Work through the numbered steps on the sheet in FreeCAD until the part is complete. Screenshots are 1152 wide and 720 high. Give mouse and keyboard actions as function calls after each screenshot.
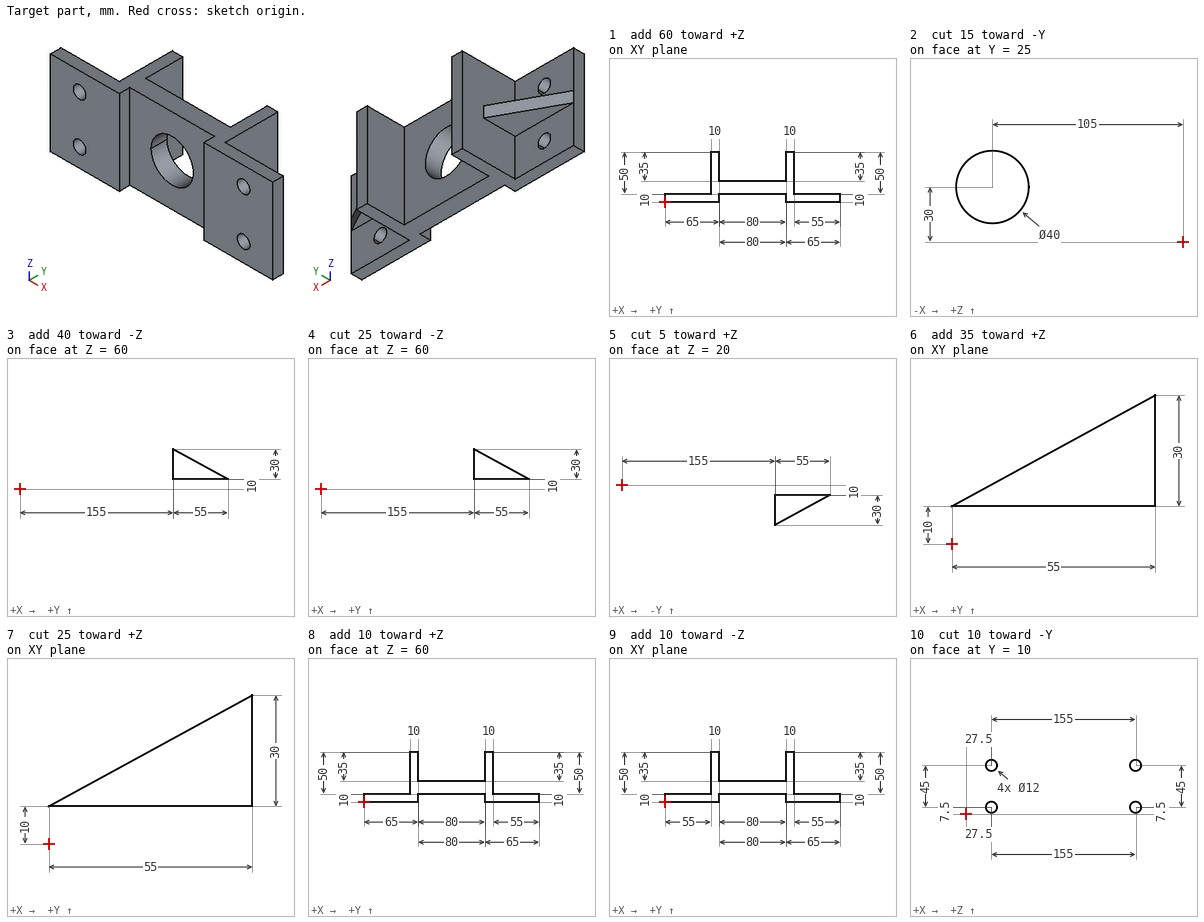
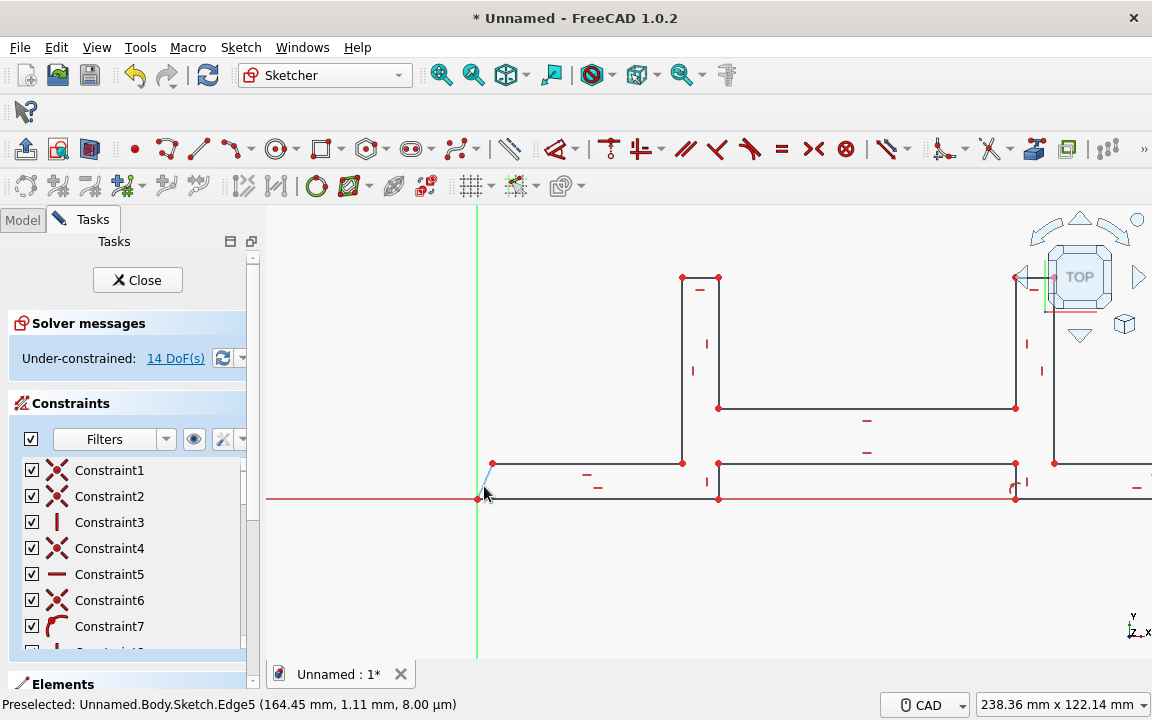
click(484, 485)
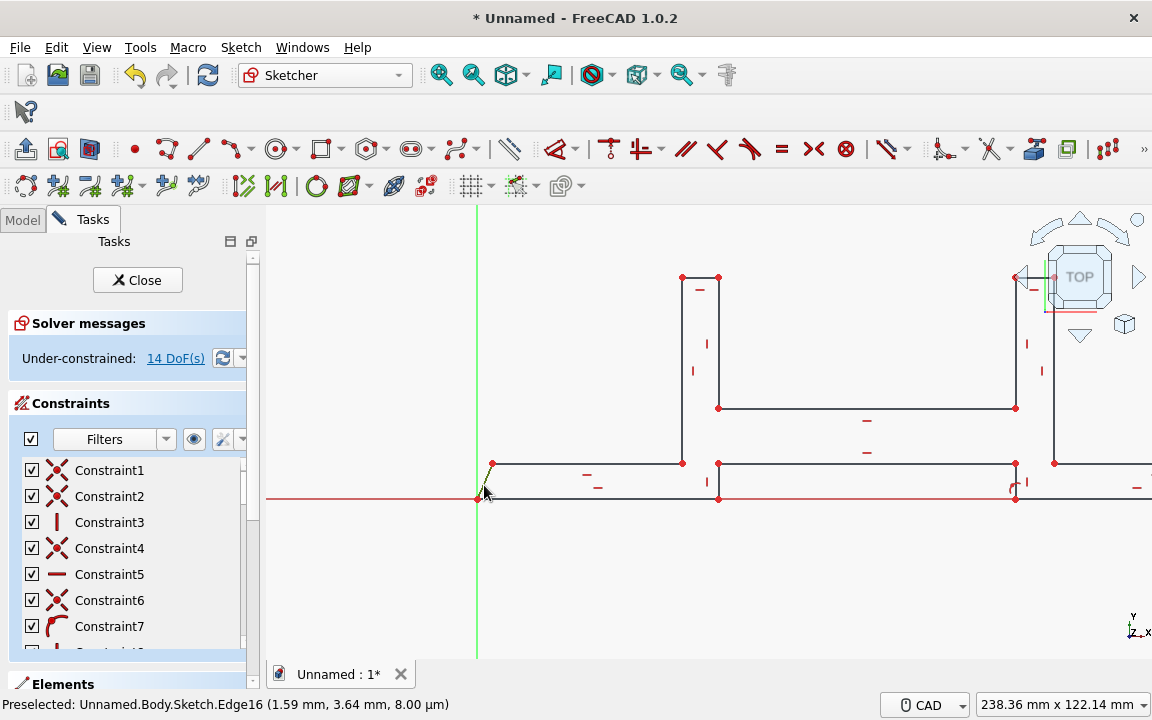
key(v)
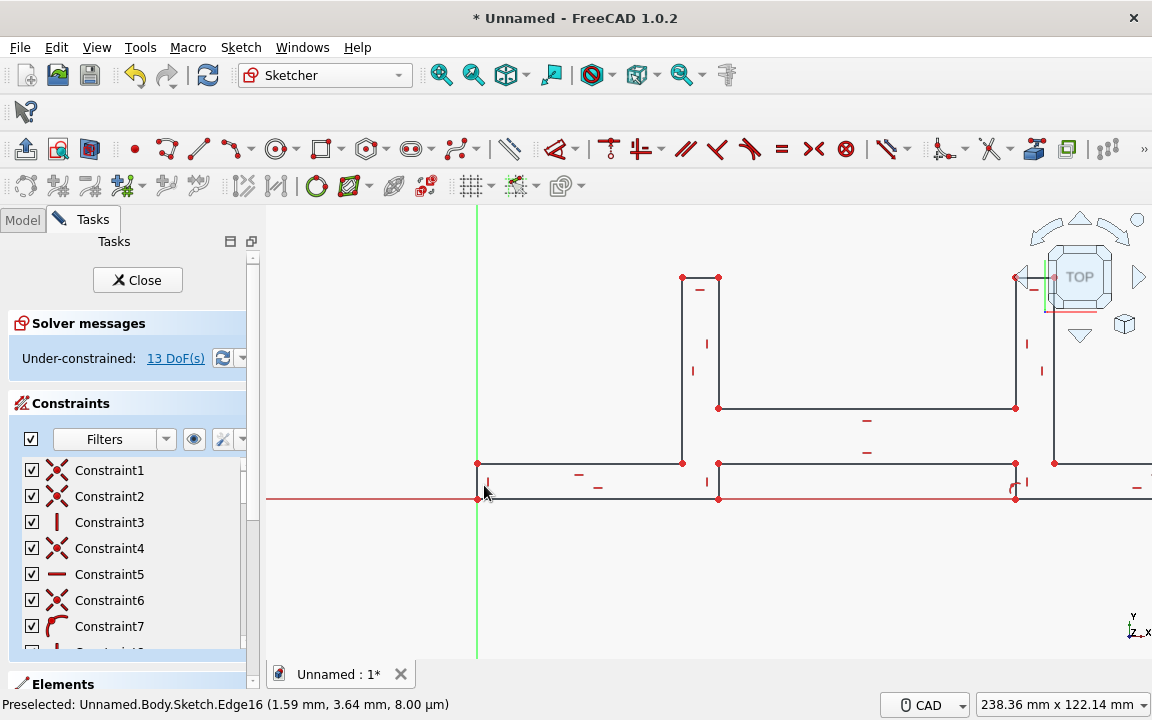
click(556, 150)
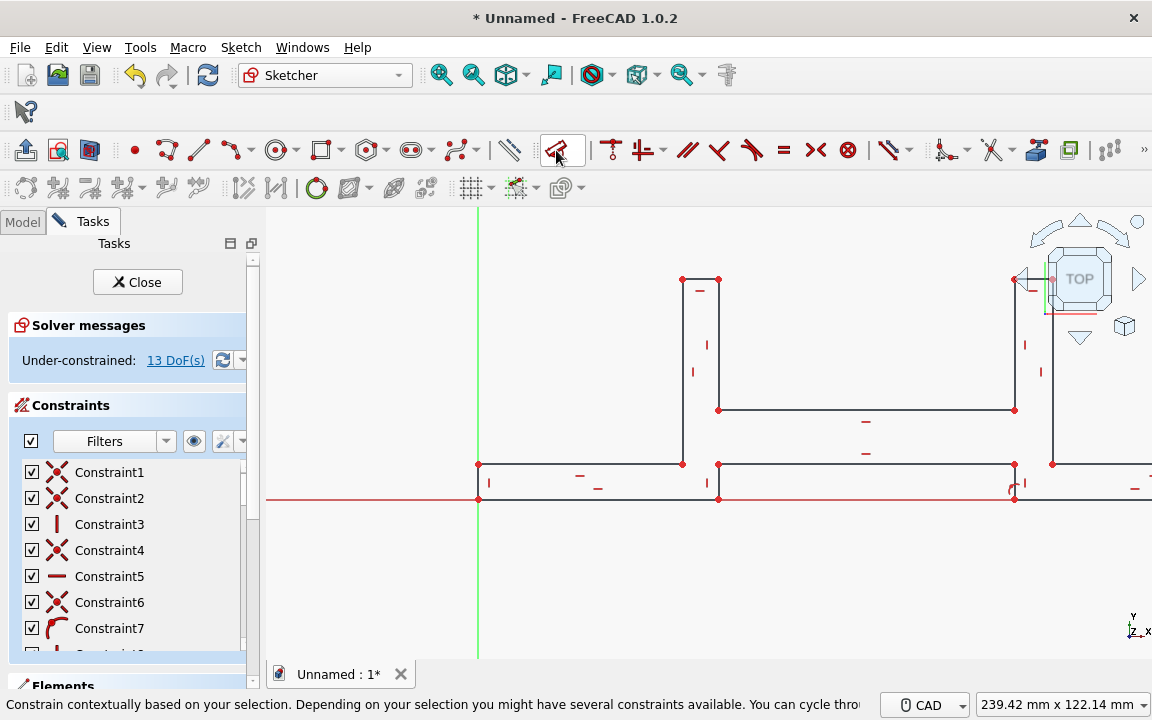
click(551, 500)
click(599, 534)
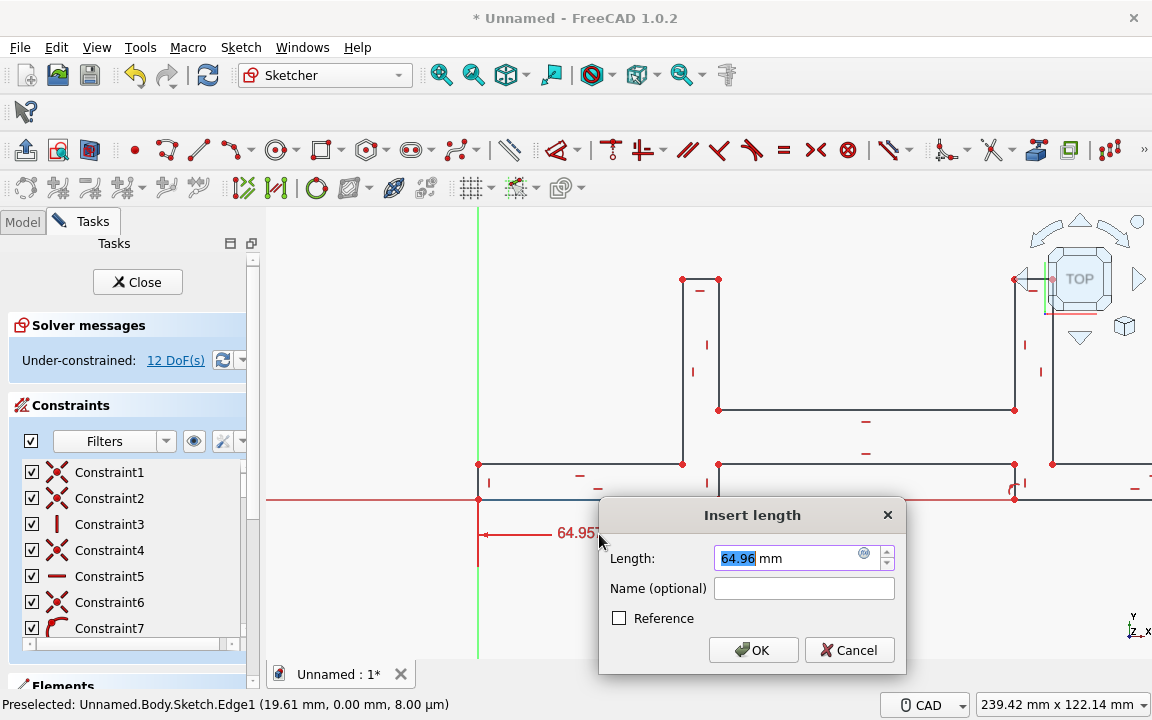
text(65)
key(Return)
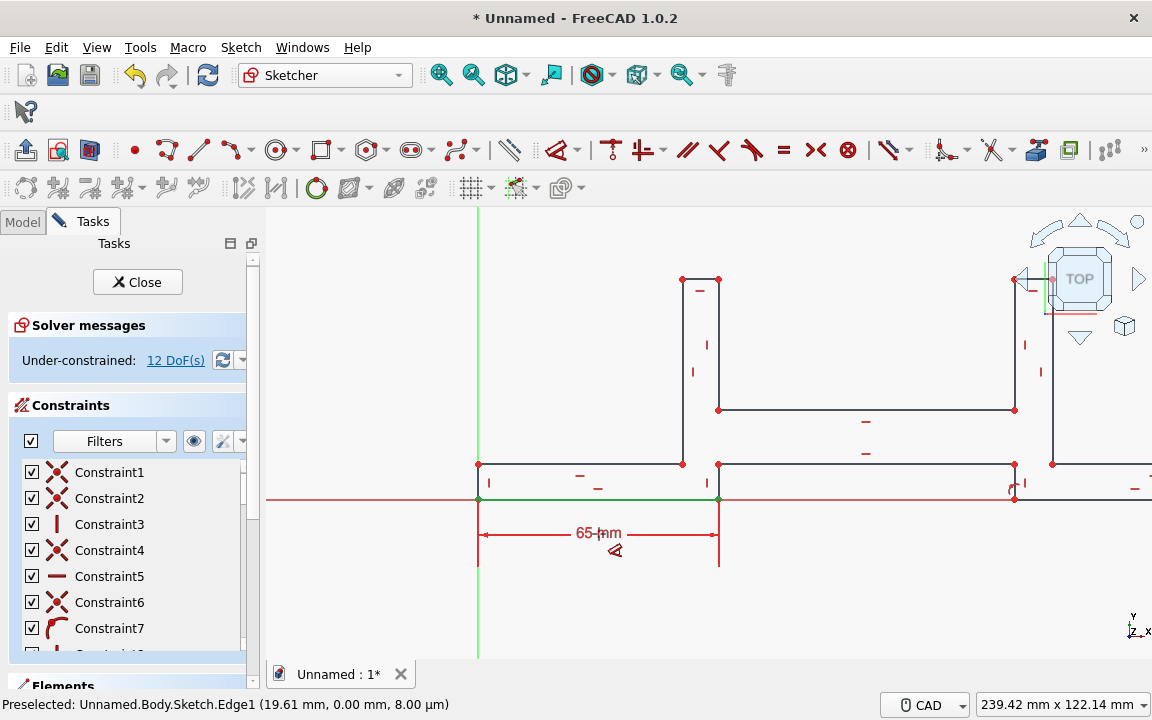
scroll(719, 489, up, 2)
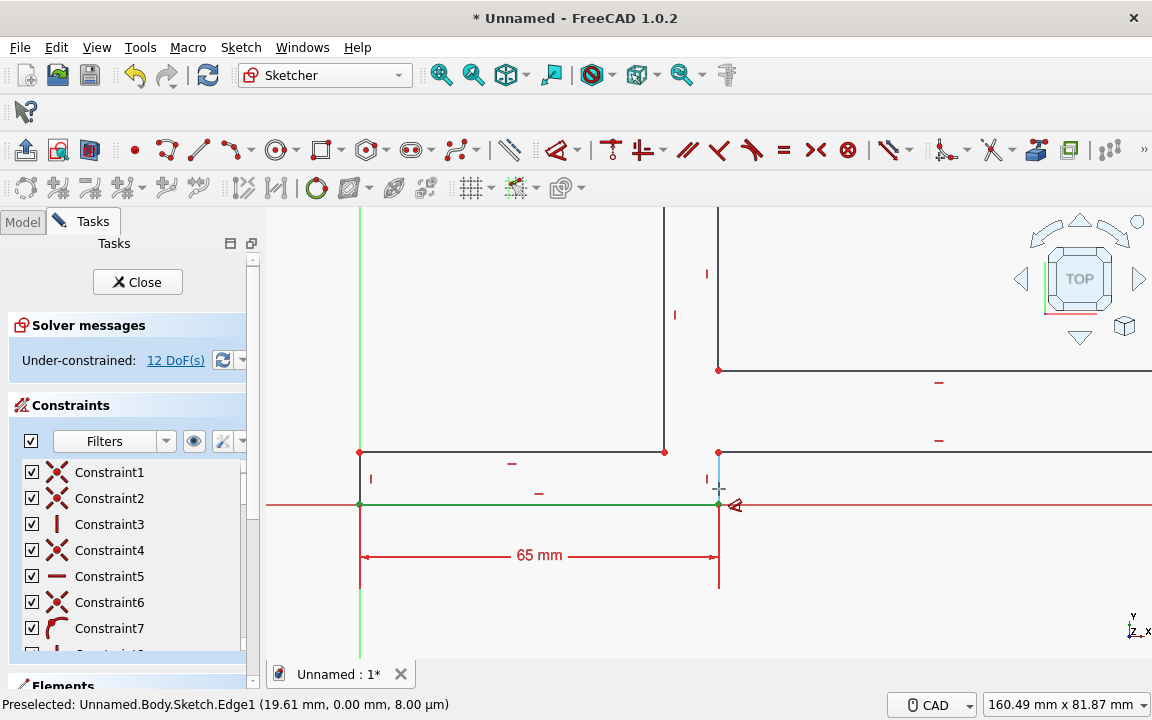
click(719, 489)
click(685, 479)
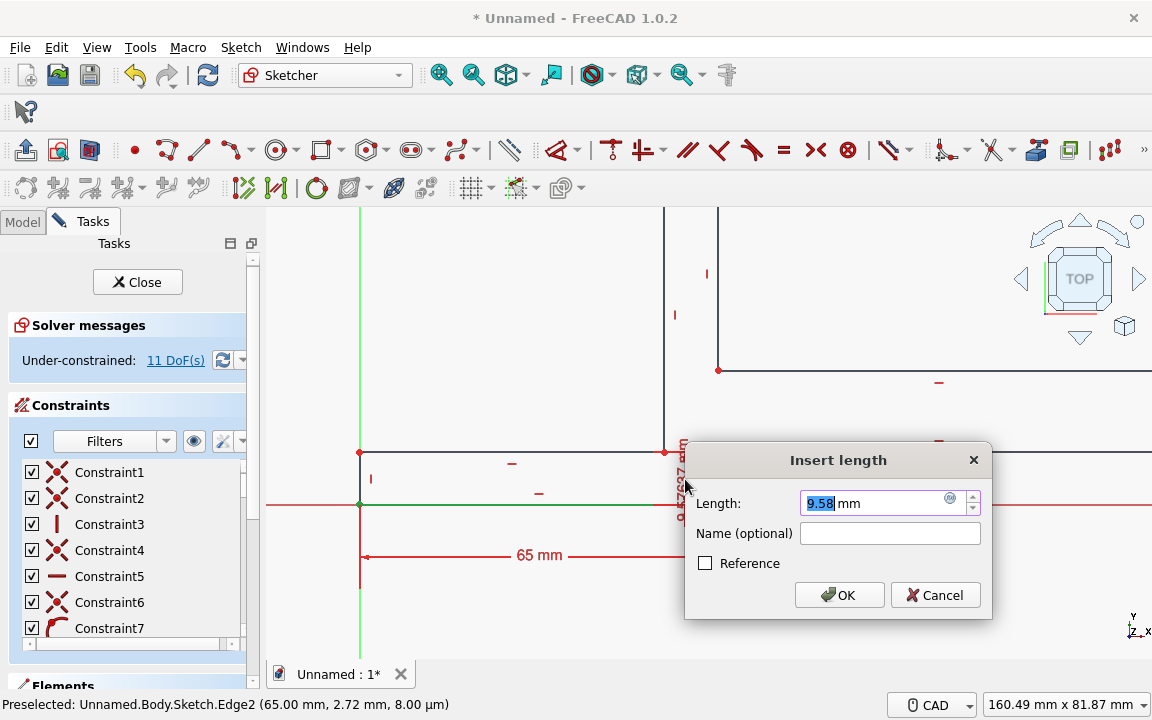
text(10)
key(Return)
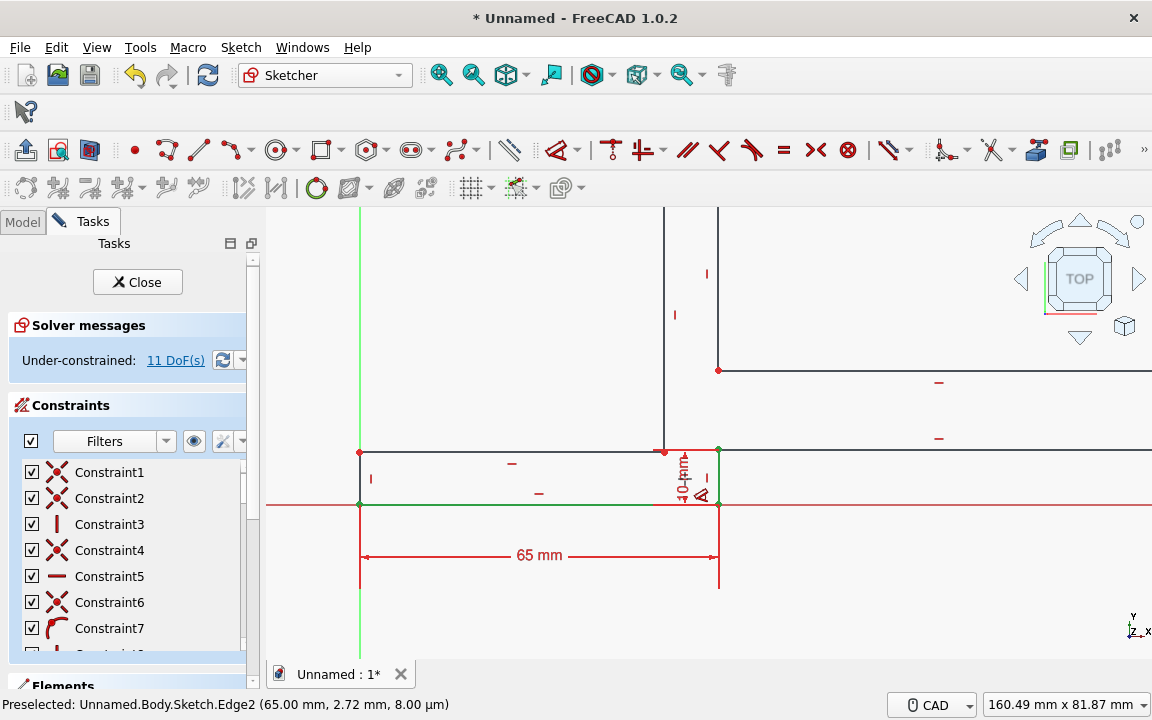
click(851, 450)
click(853, 484)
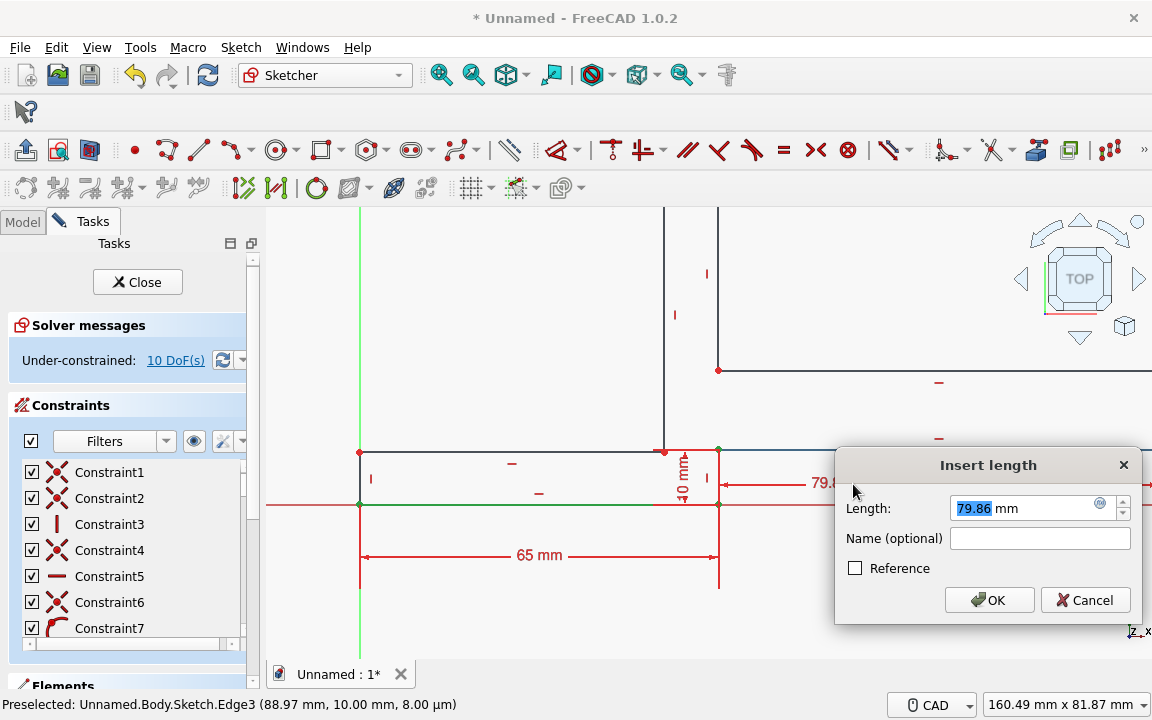
text(80)
key(Return)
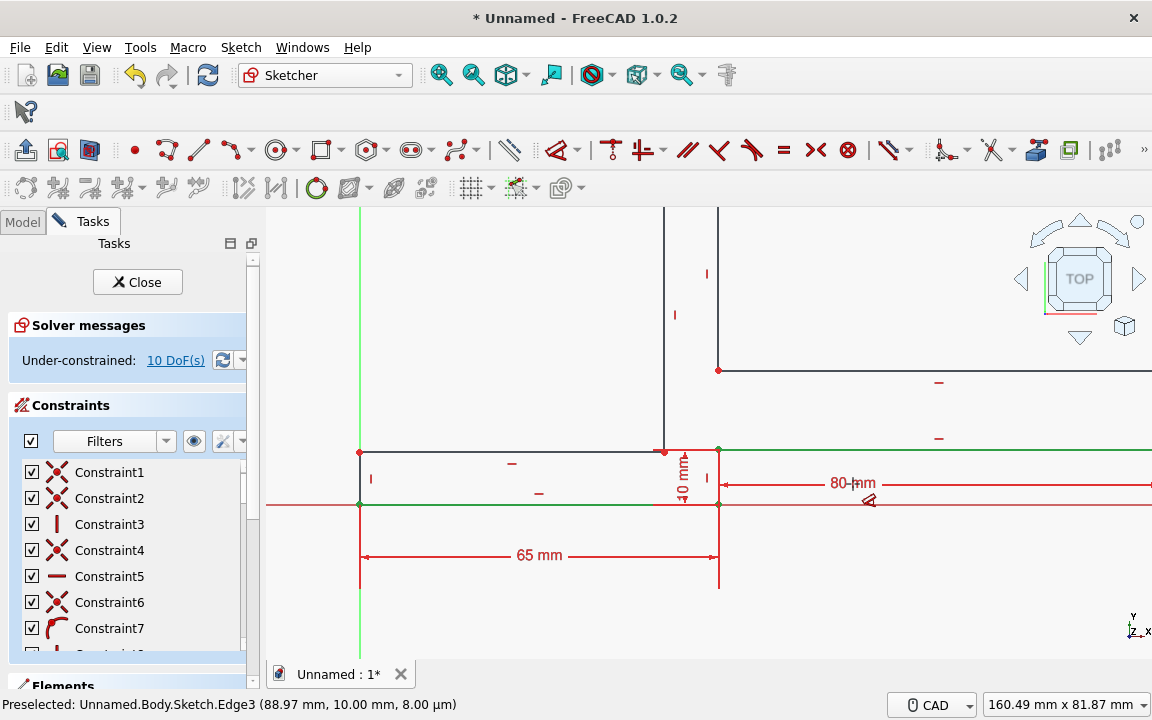
scroll(397, 509, down, 4)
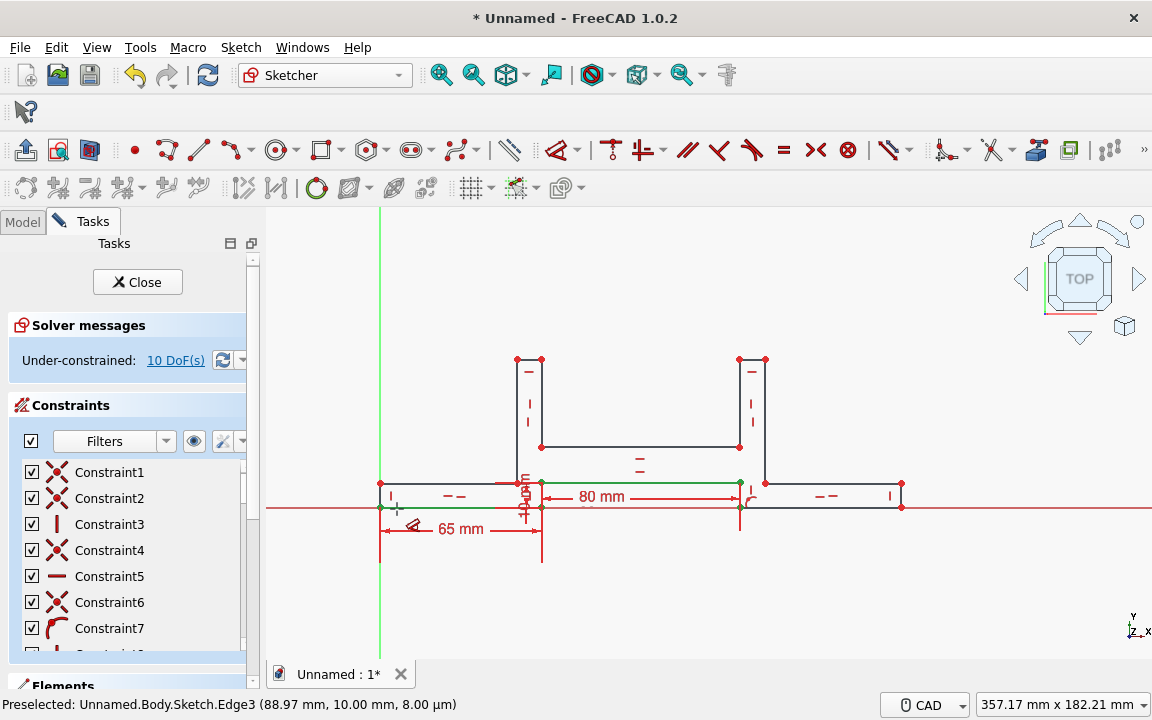
click(788, 508)
click(821, 542)